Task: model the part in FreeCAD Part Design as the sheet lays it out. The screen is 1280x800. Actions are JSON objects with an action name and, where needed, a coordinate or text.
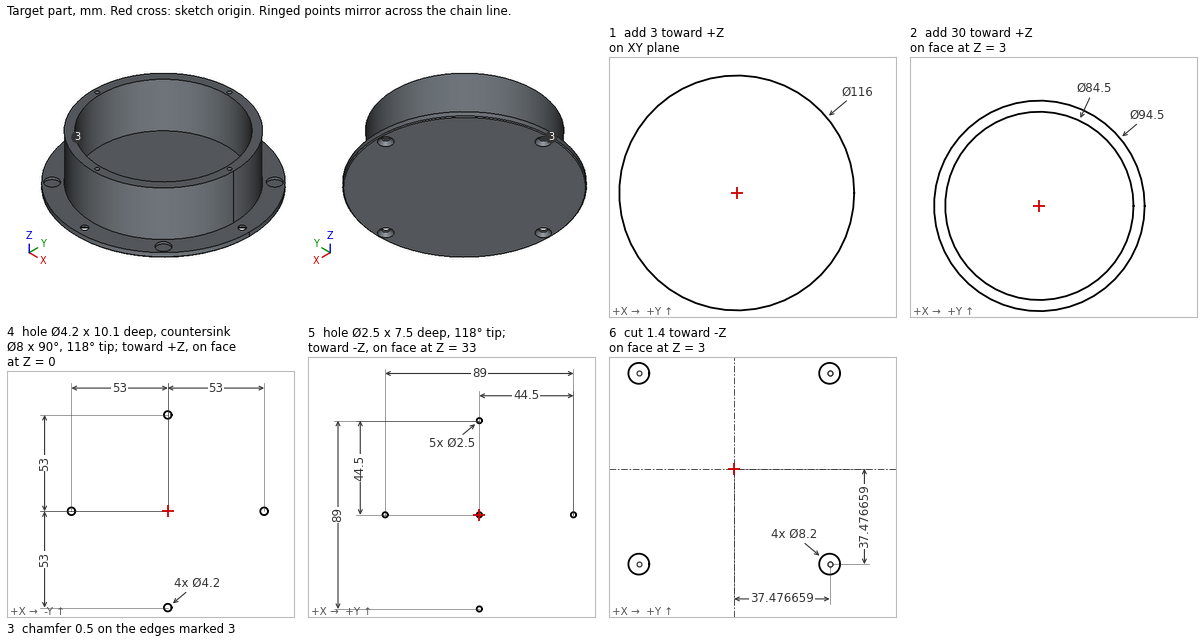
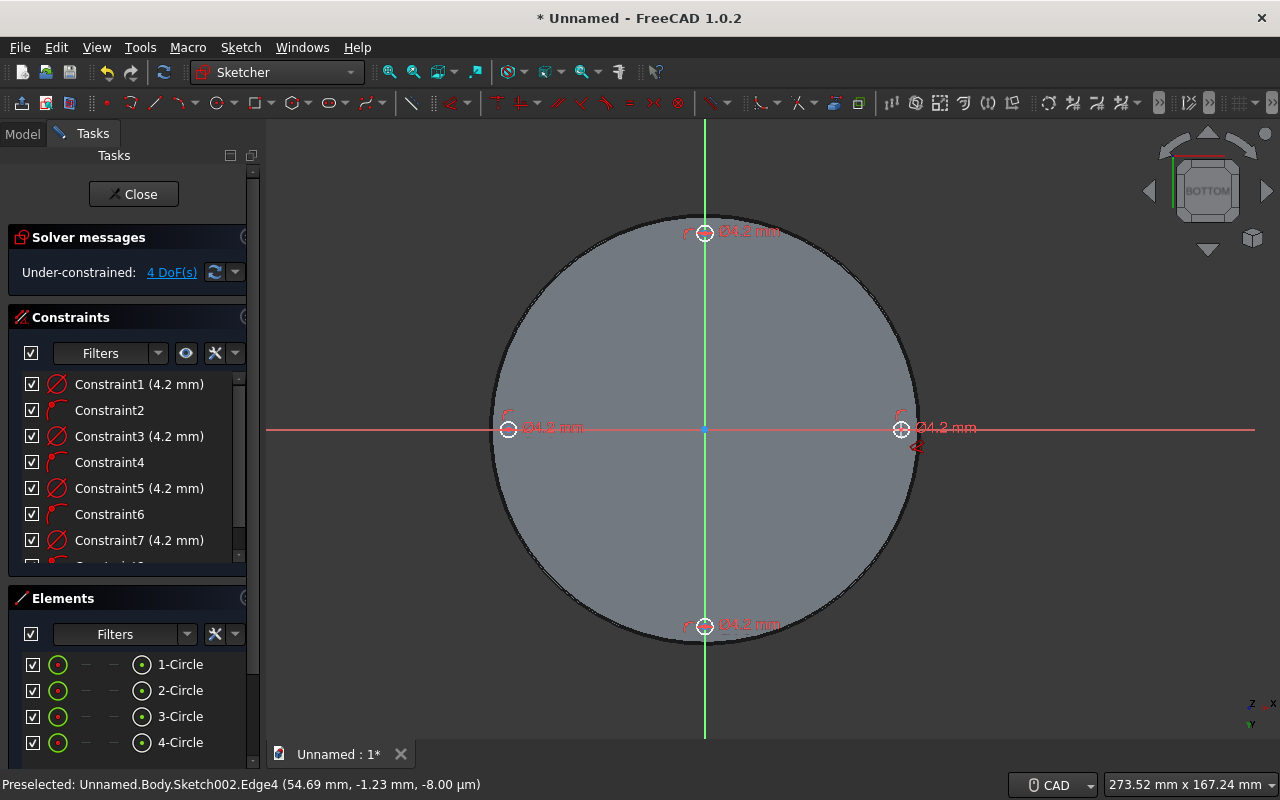
{"action": "left_click", "coordinate": [705, 627]}
{"action": "left_click", "coordinate": [739, 528]}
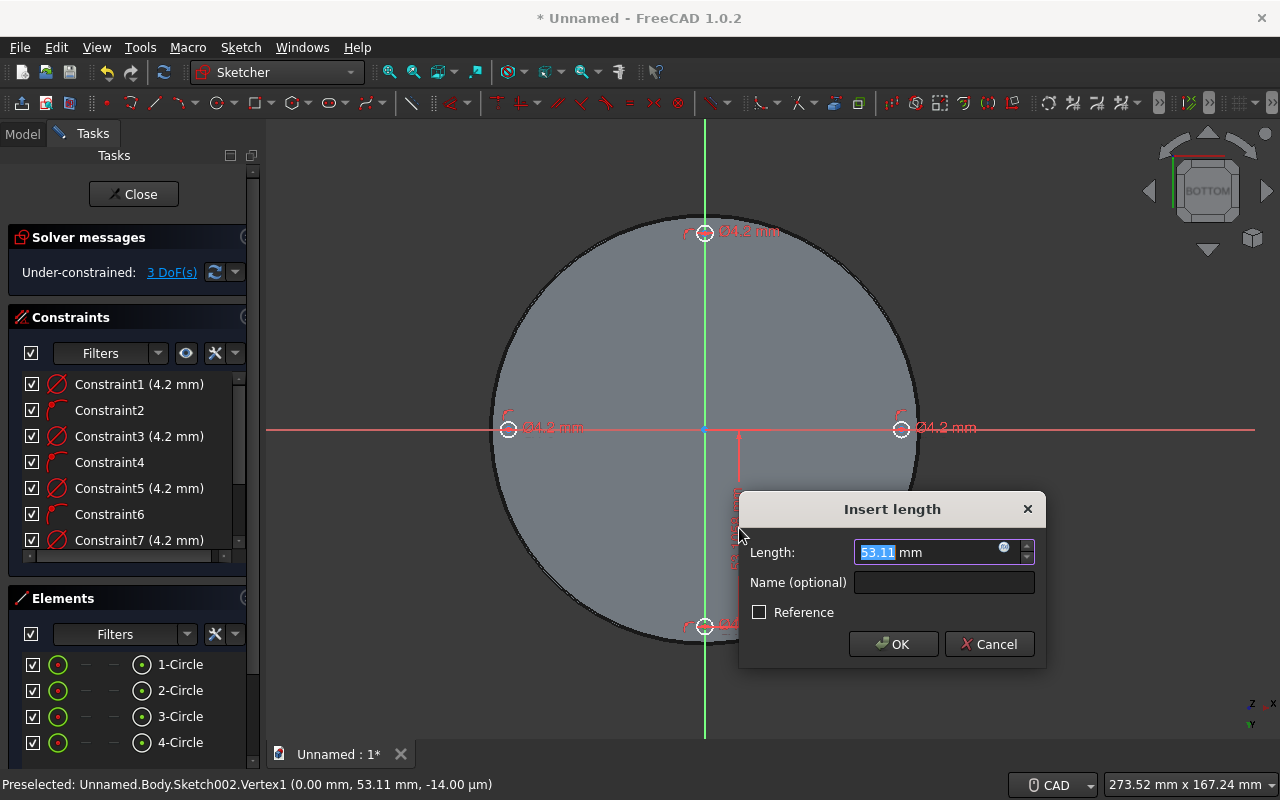
{"action": "type", "text": "53"}
{"action": "key", "text": "Return"}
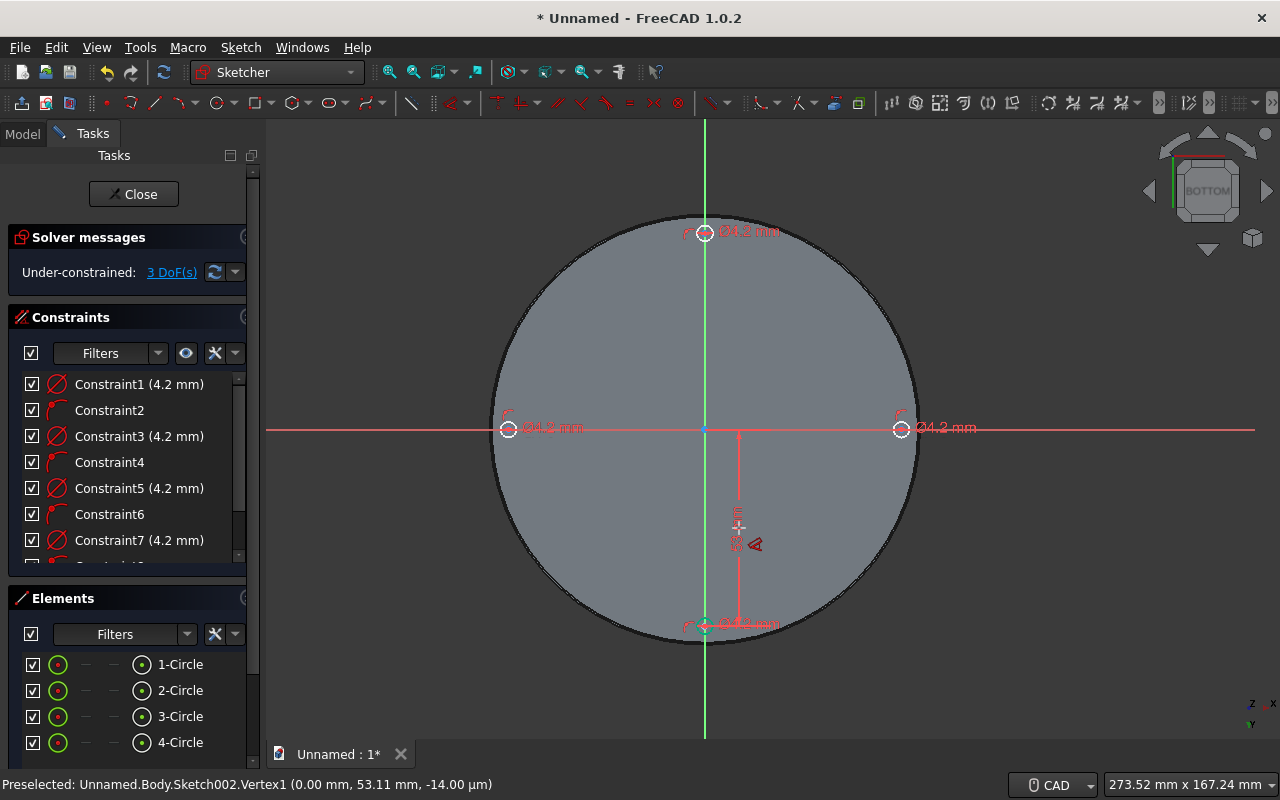
{"action": "left_click", "coordinate": [509, 430]}
{"action": "left_click", "coordinate": [607, 464]}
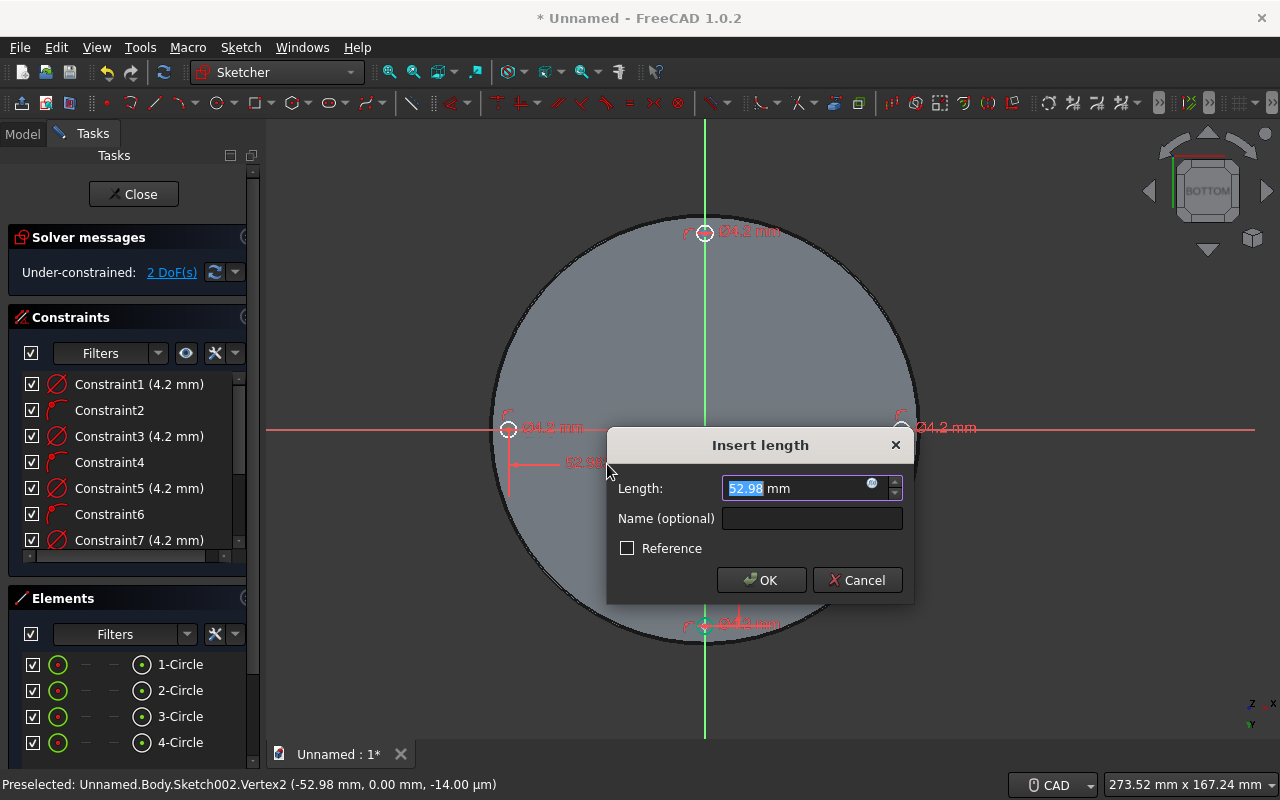
{"action": "type", "text": "53"}
{"action": "key", "text": "Return"}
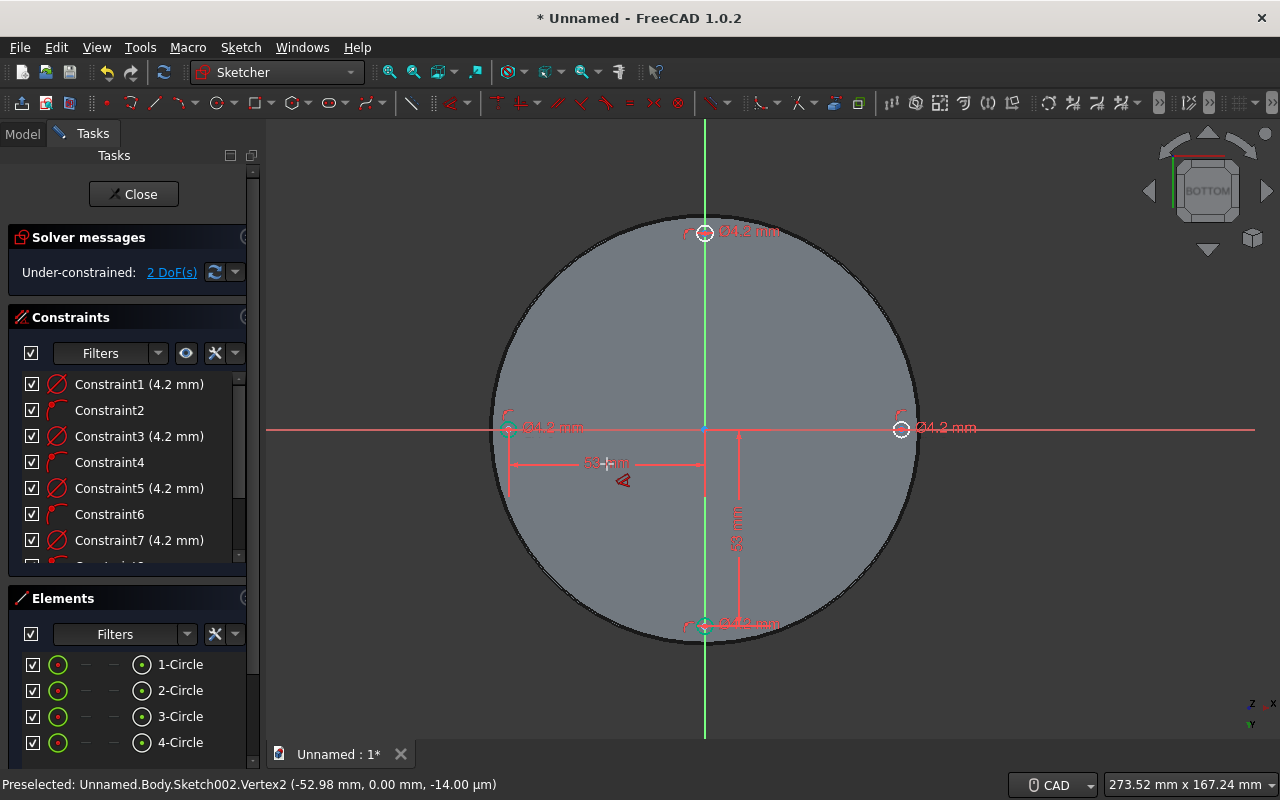
{"action": "left_click", "coordinate": [705, 233]}
{"action": "left_click", "coordinate": [739, 332]}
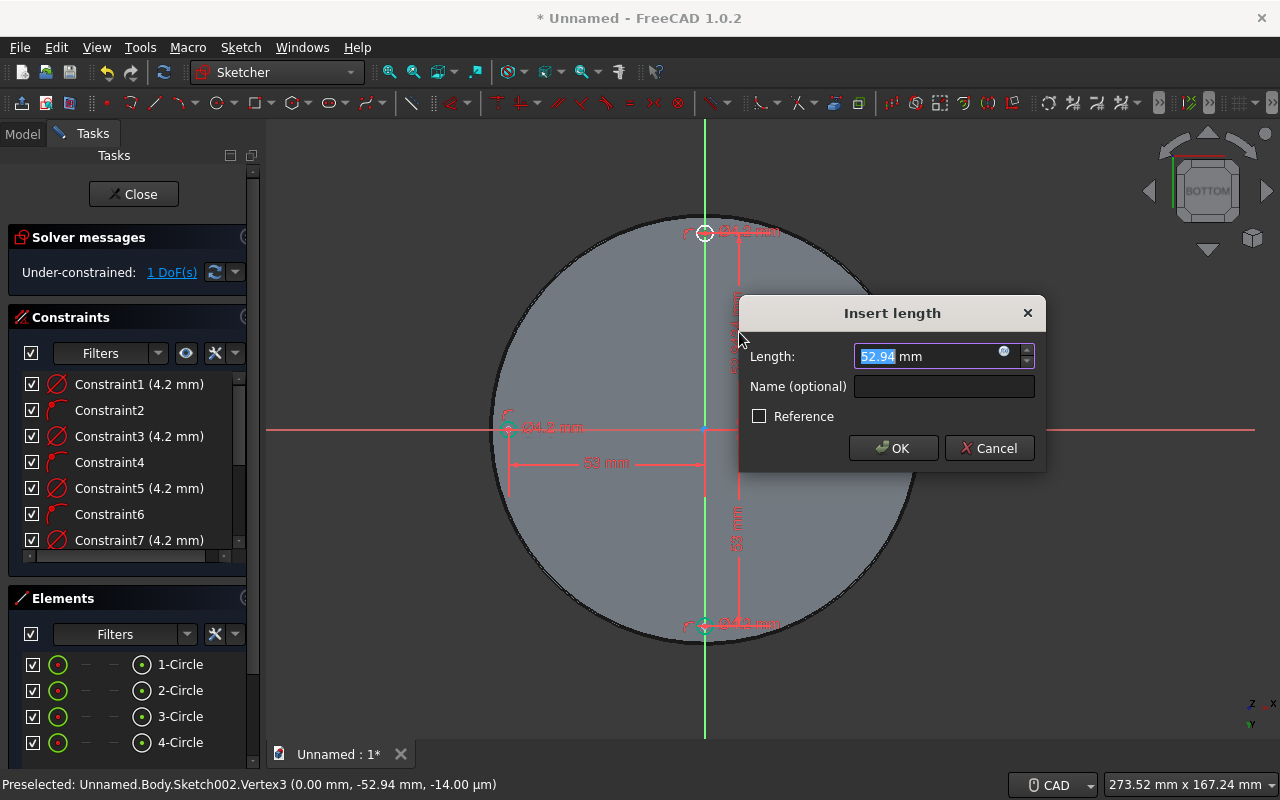
{"action": "type", "text": "53"}
{"action": "key", "text": "Return"}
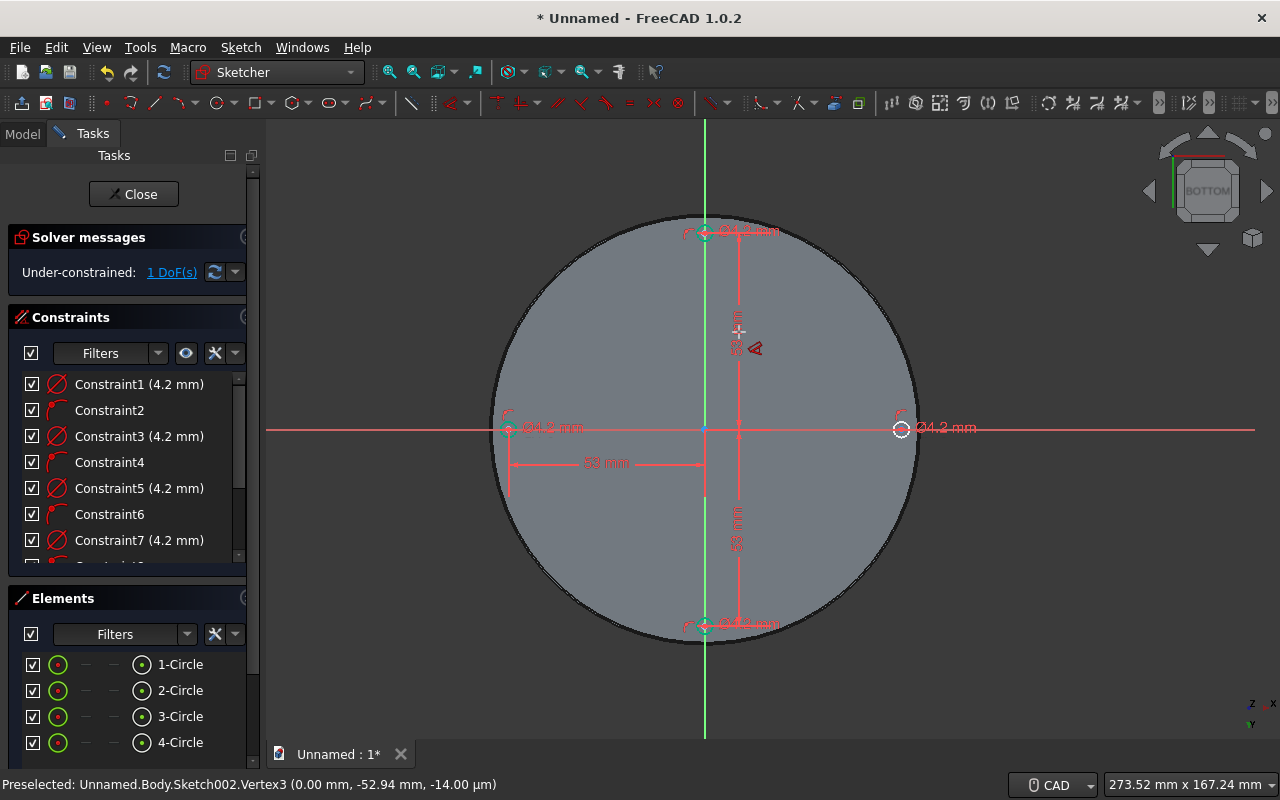
{"action": "left_click", "coordinate": [901, 430]}
{"action": "left_click", "coordinate": [803, 464]}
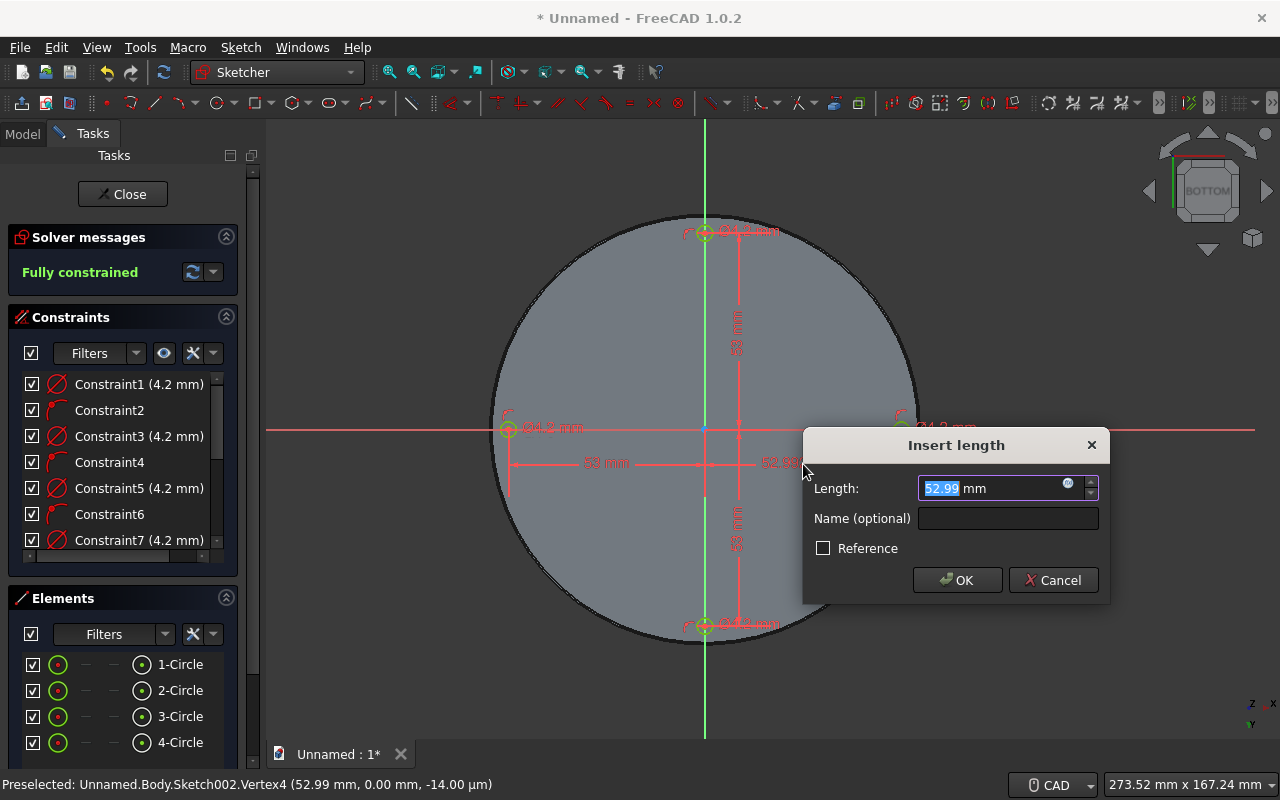
{"action": "type", "text": "53"}
{"action": "key", "text": "Return"}
{"action": "key", "text": "Escape"}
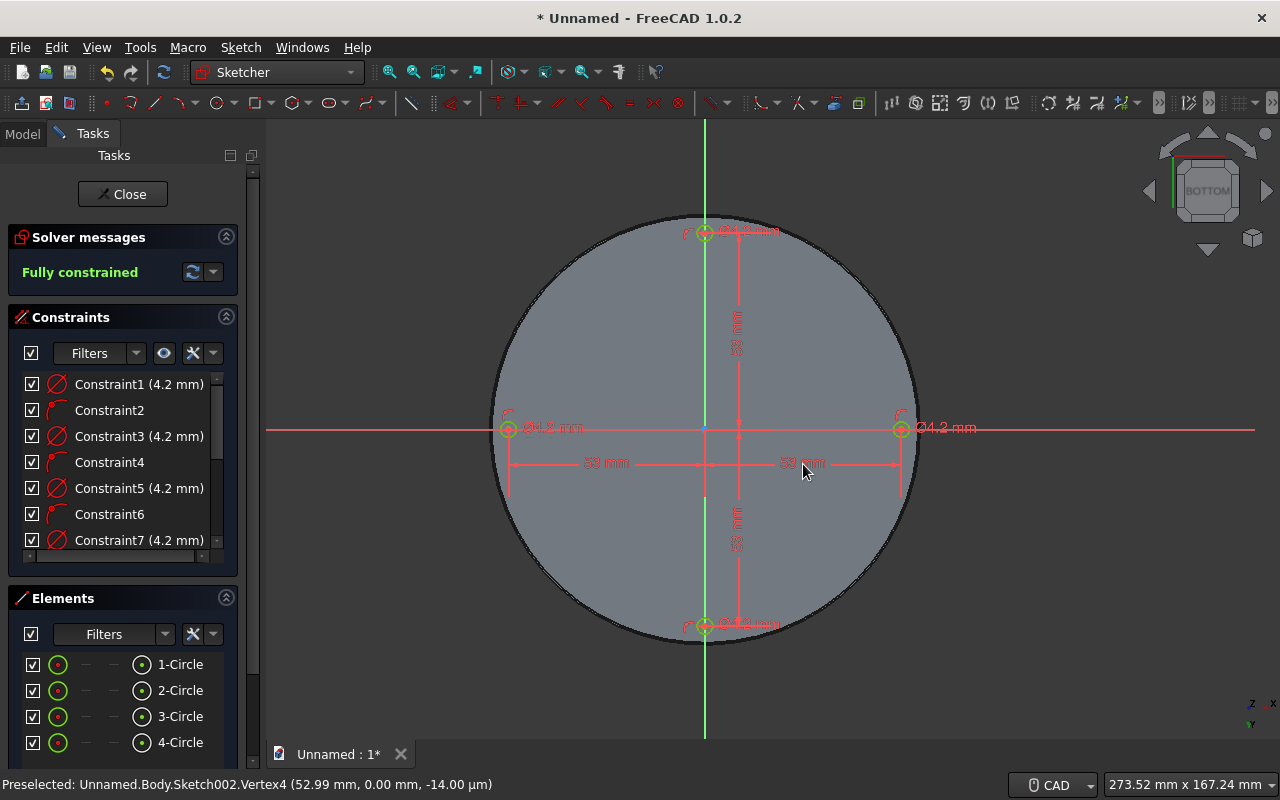
{"action": "left_click", "coordinate": [123, 194]}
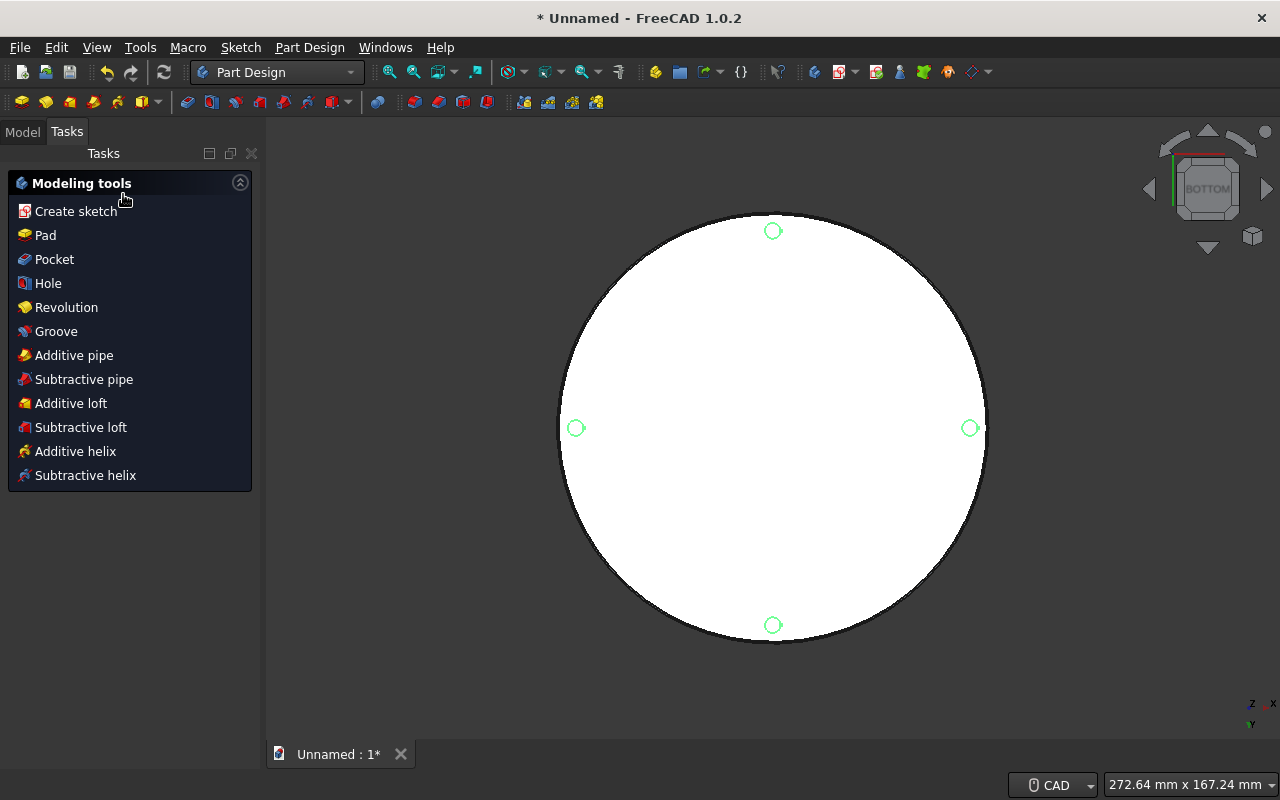
{"action": "left_click", "coordinate": [212, 102]}